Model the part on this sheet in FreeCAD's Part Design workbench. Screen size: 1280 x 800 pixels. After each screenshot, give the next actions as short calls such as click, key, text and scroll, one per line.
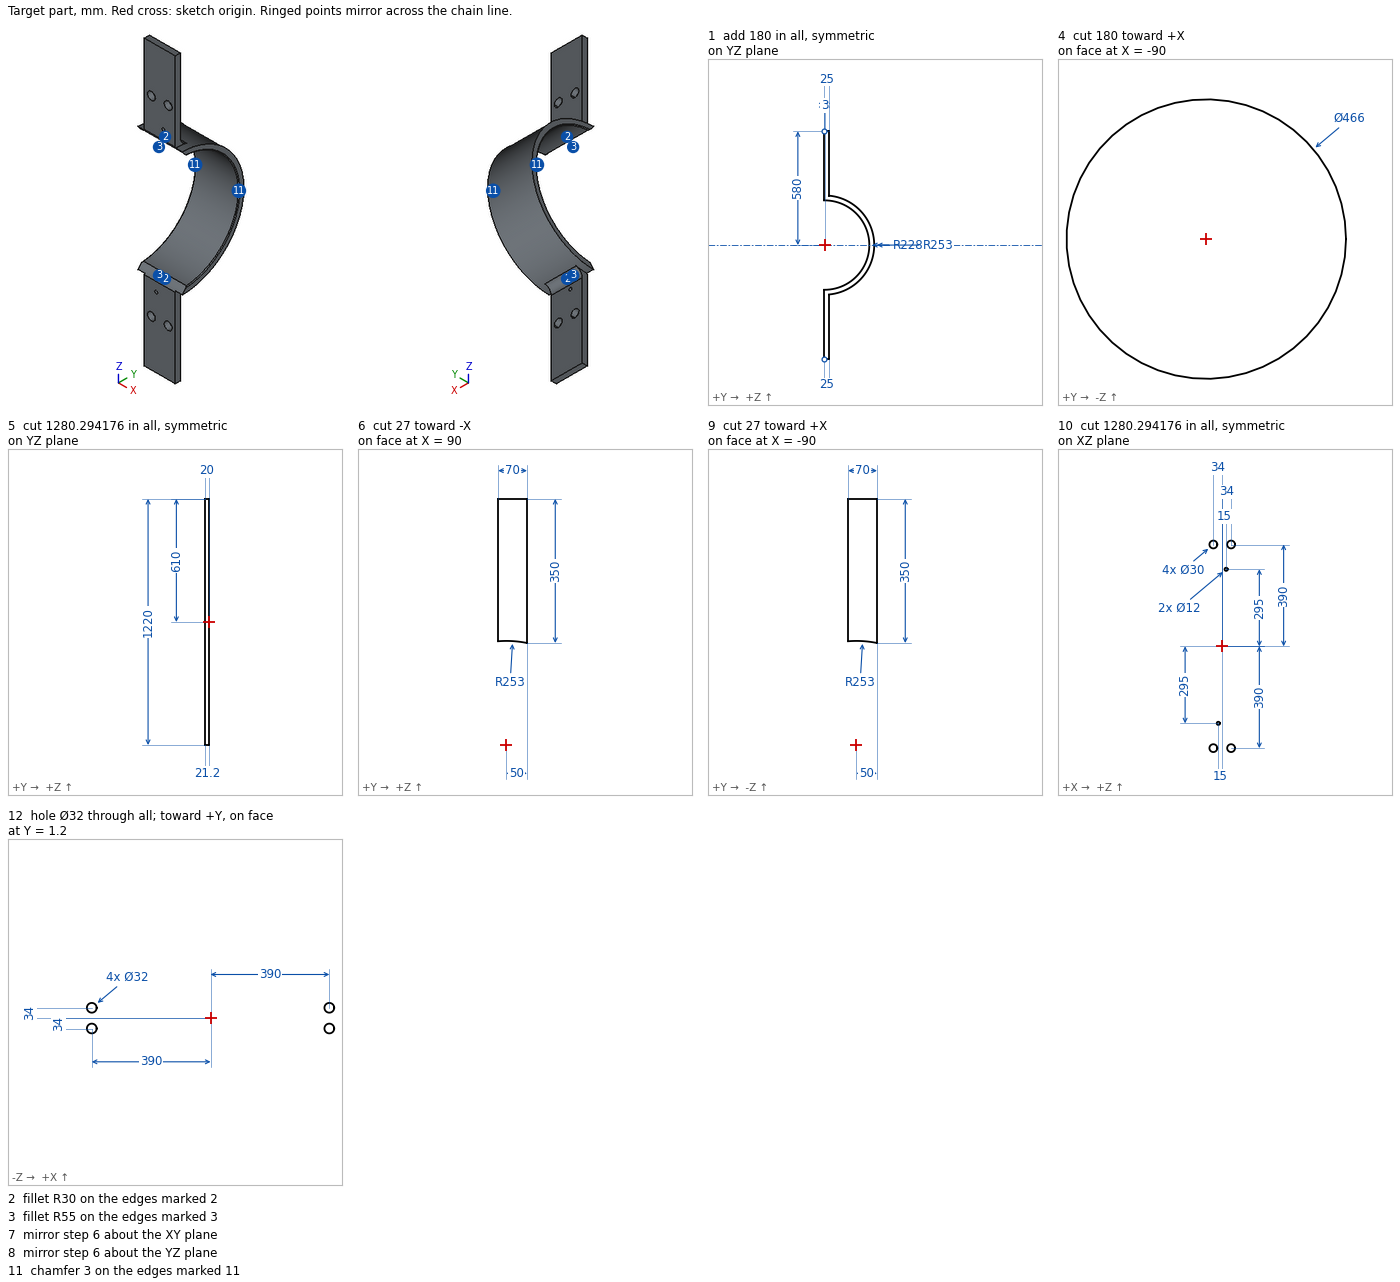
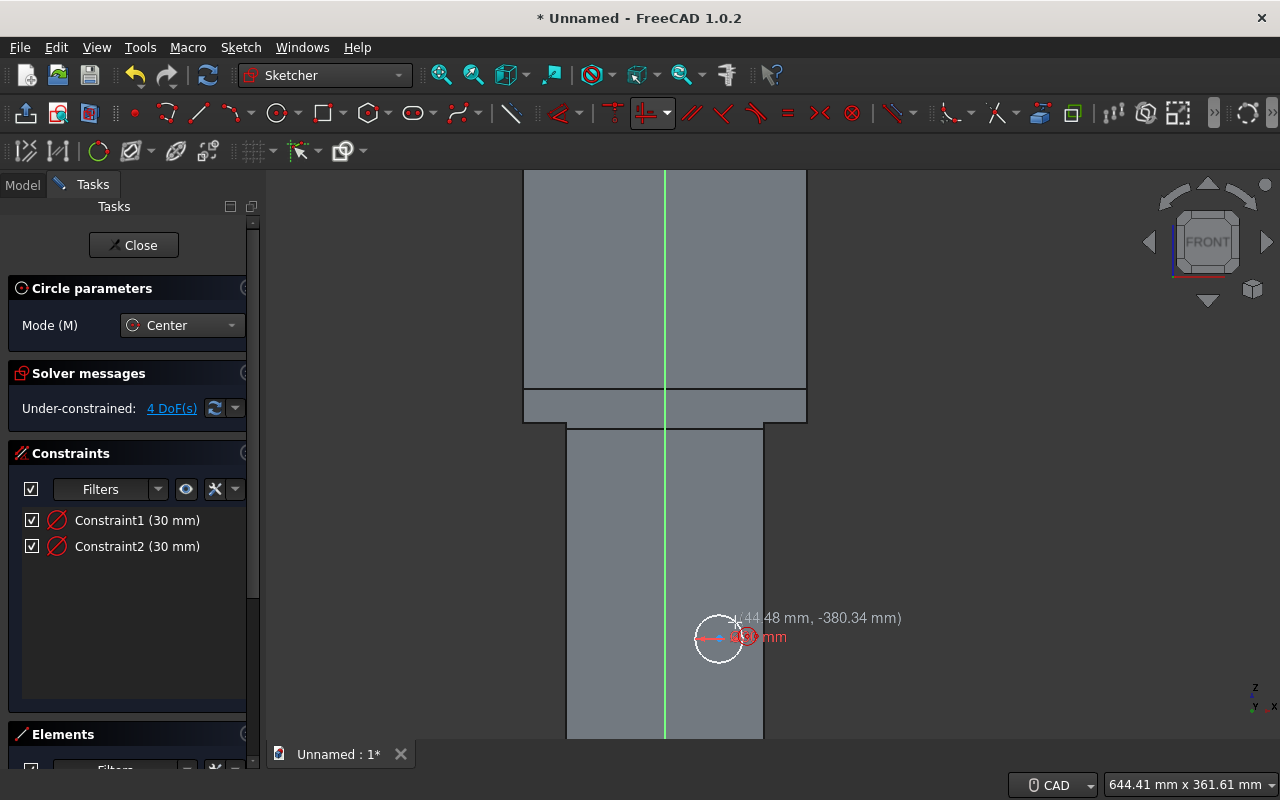
scroll(722, 640, down, 6)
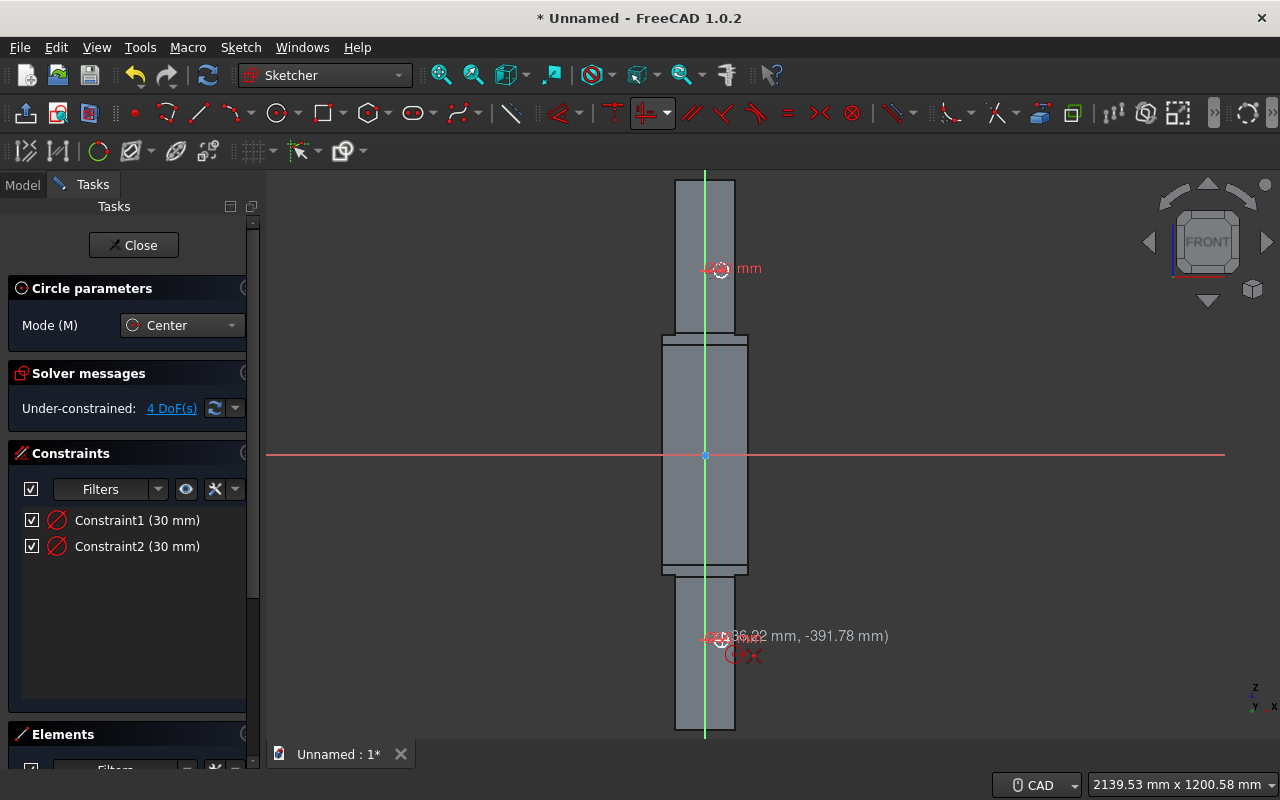
scroll(689, 270, up, 6)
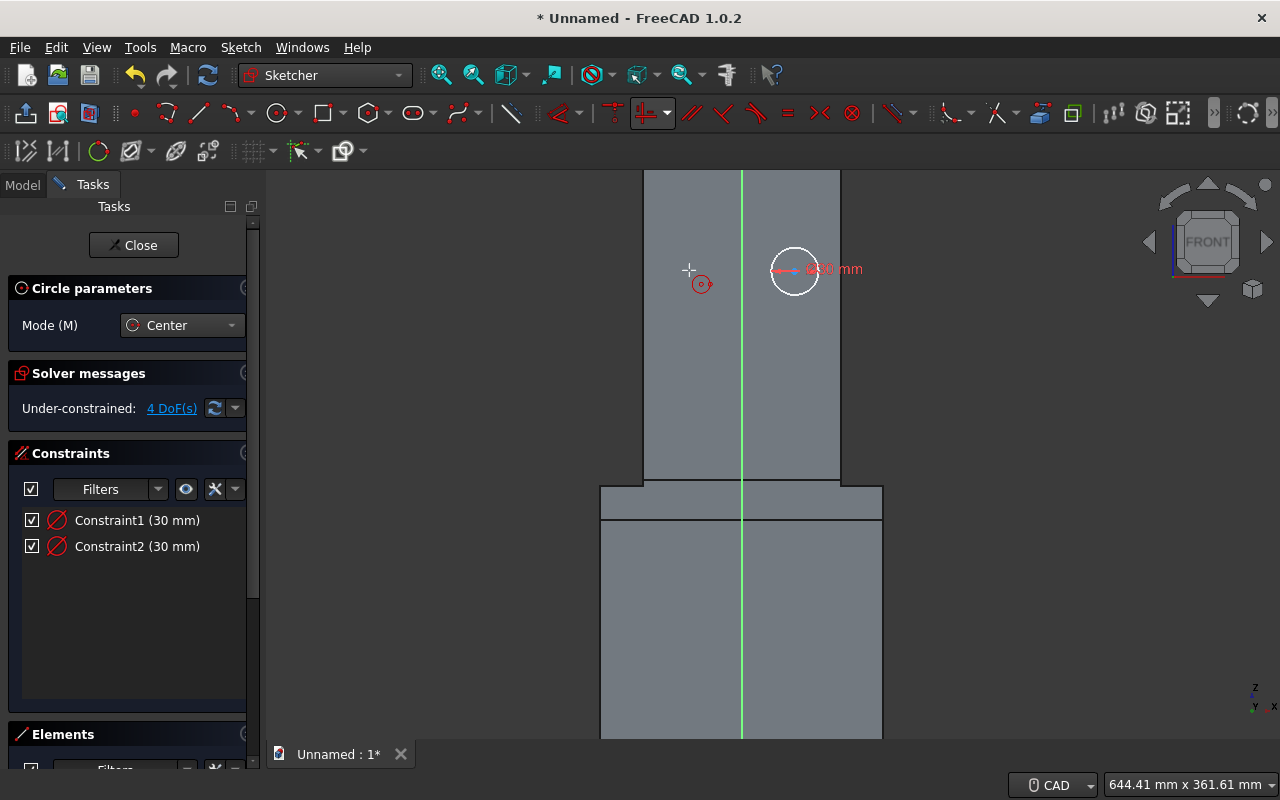
click(688, 271)
move(705, 254)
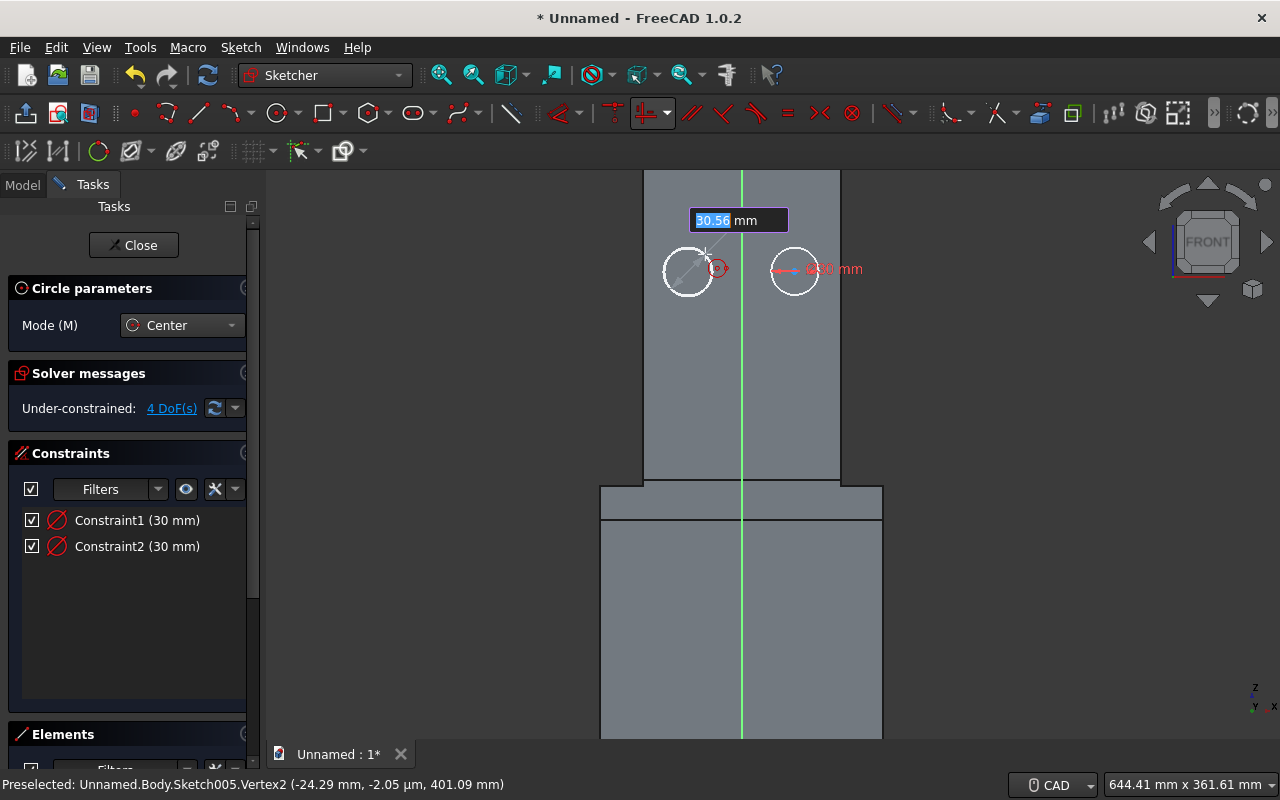
text(30)
key(Return)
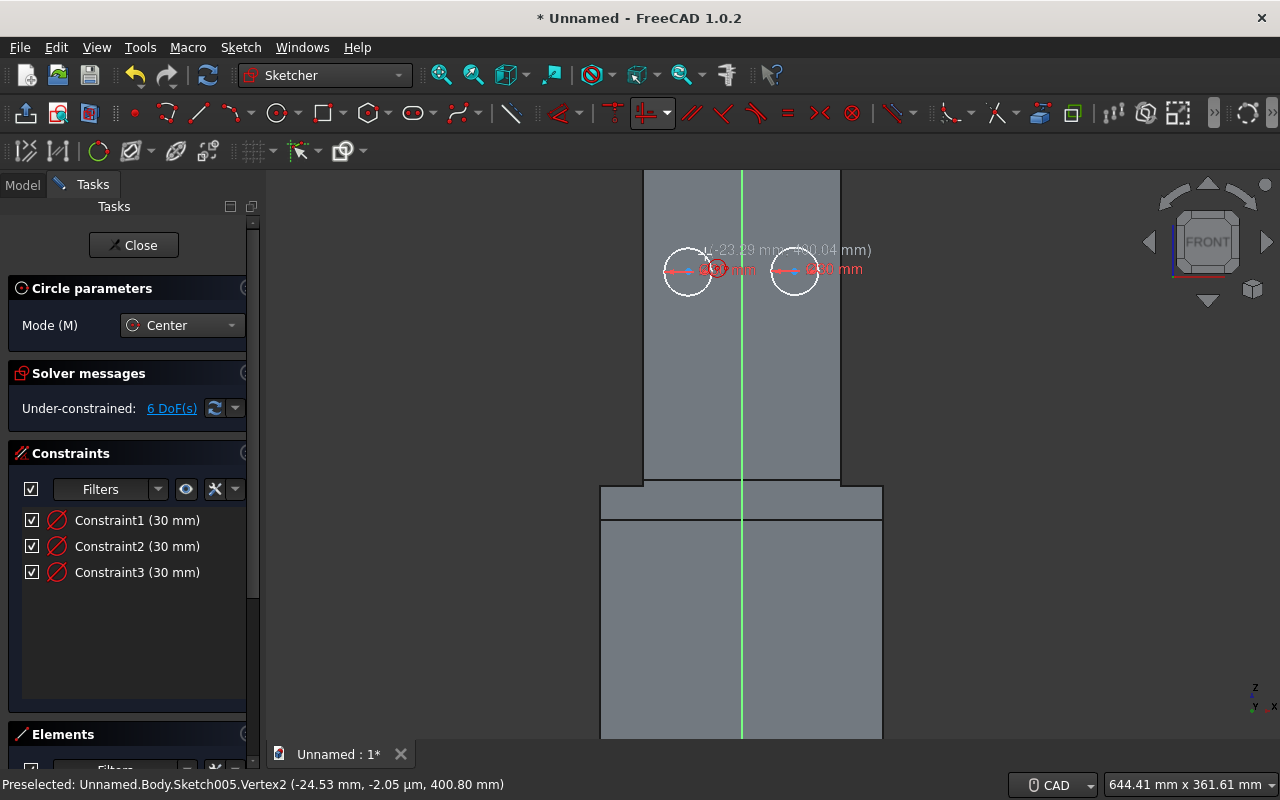
scroll(688, 269, down, 6)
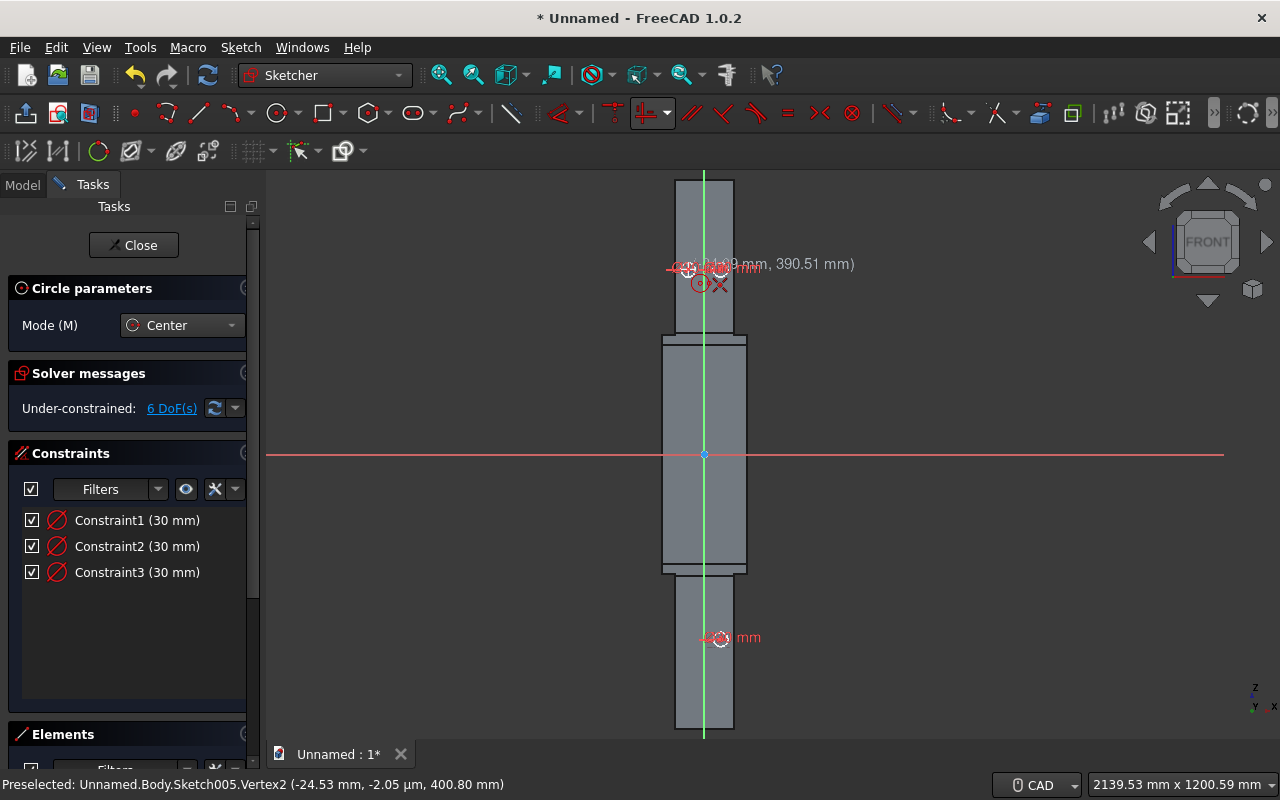
scroll(688, 639, up, 6)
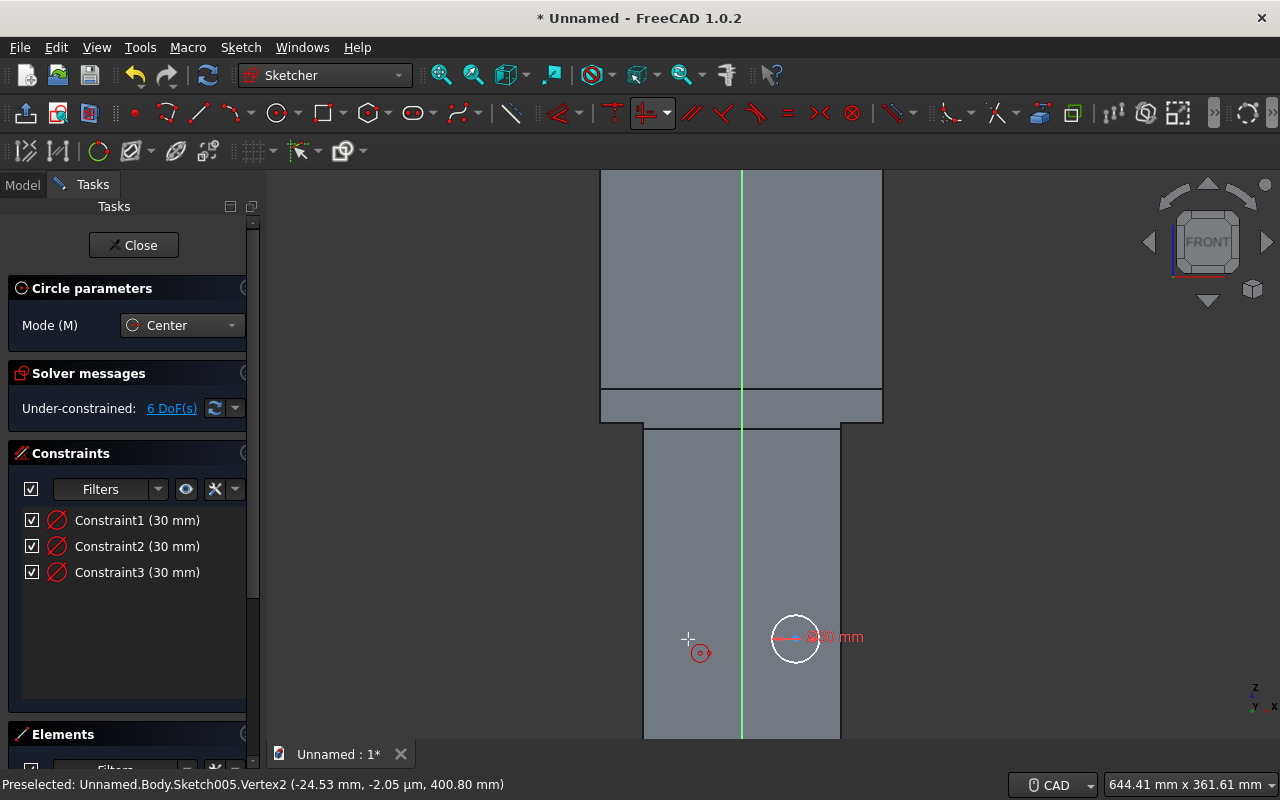
click(688, 638)
move(705, 622)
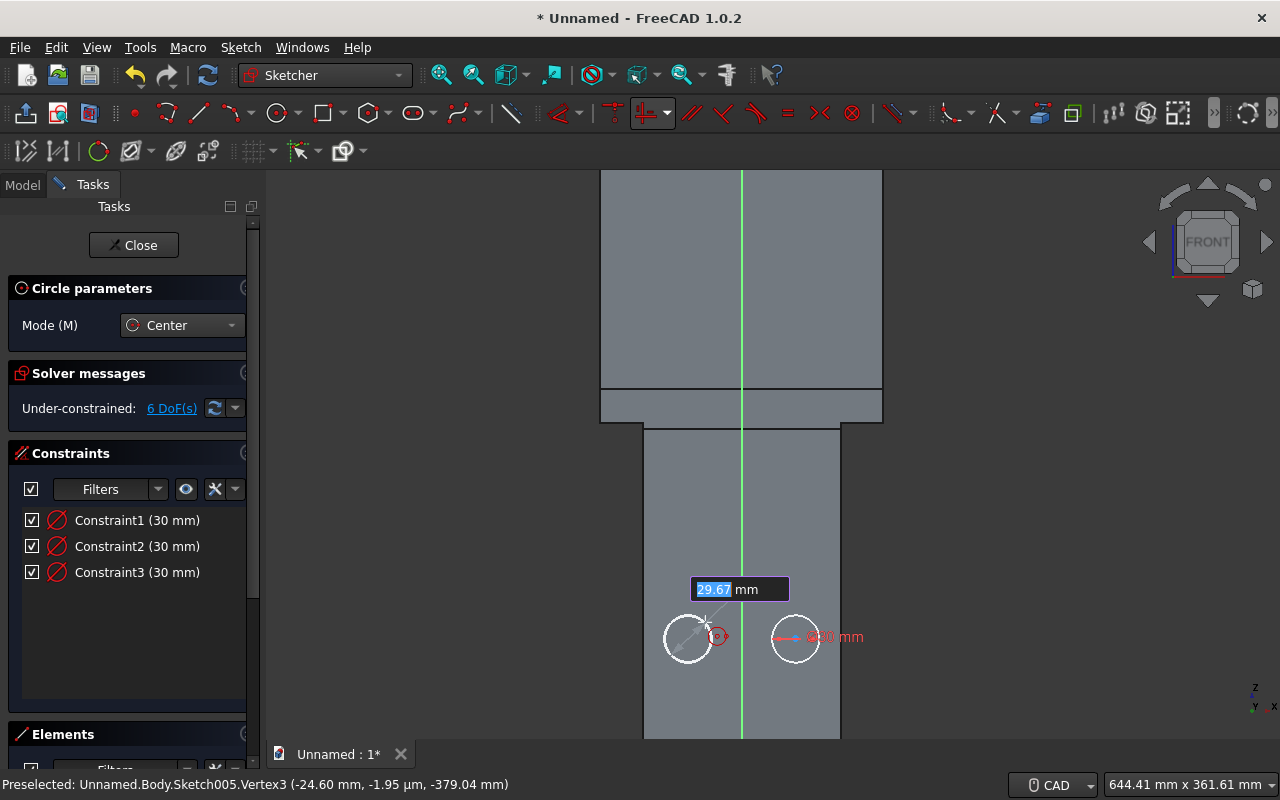
text(30)
key(Return)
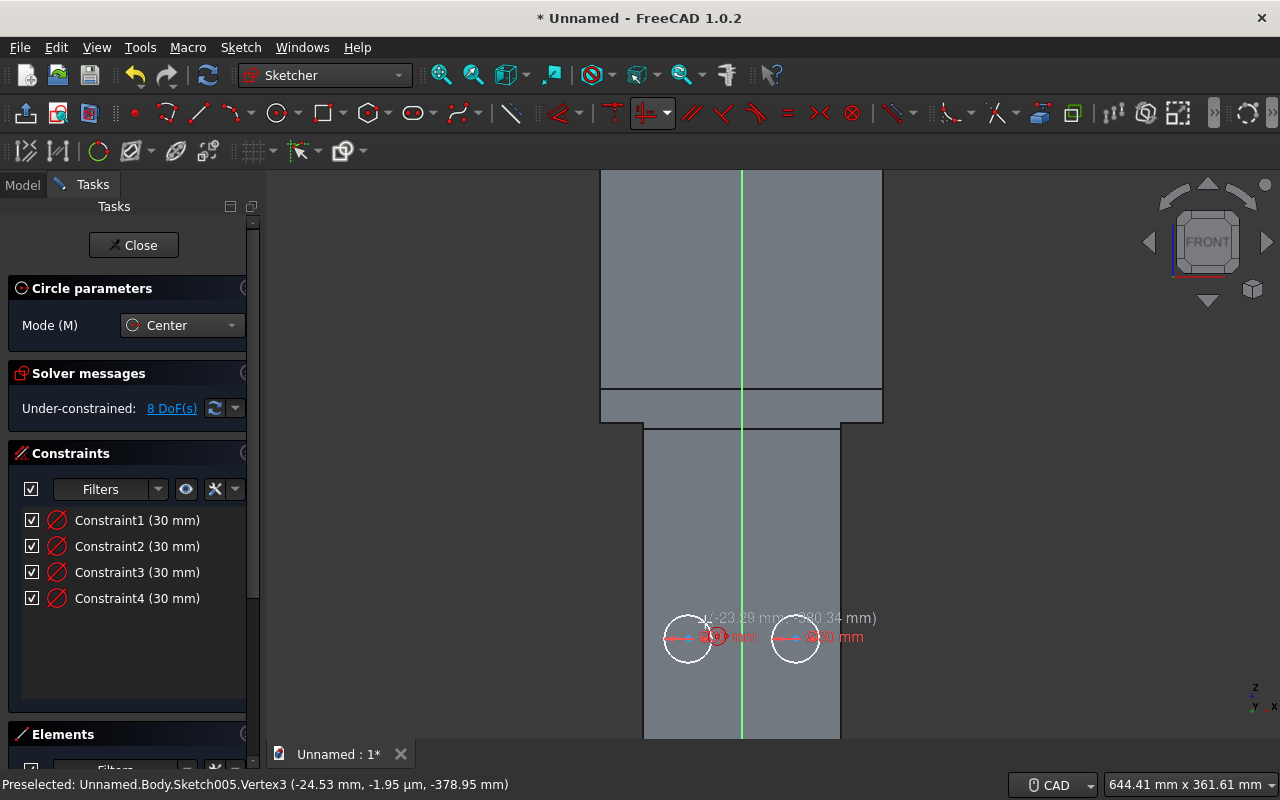
scroll(688, 640, down, 6)